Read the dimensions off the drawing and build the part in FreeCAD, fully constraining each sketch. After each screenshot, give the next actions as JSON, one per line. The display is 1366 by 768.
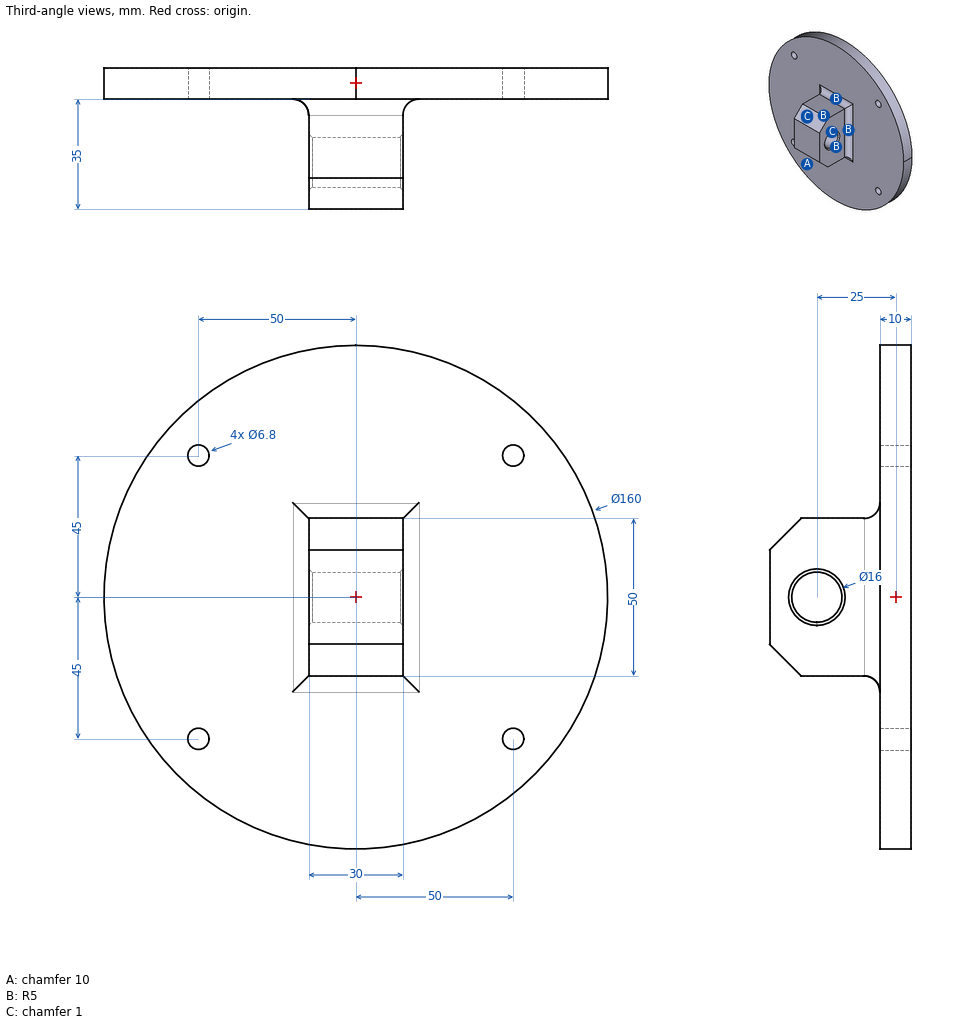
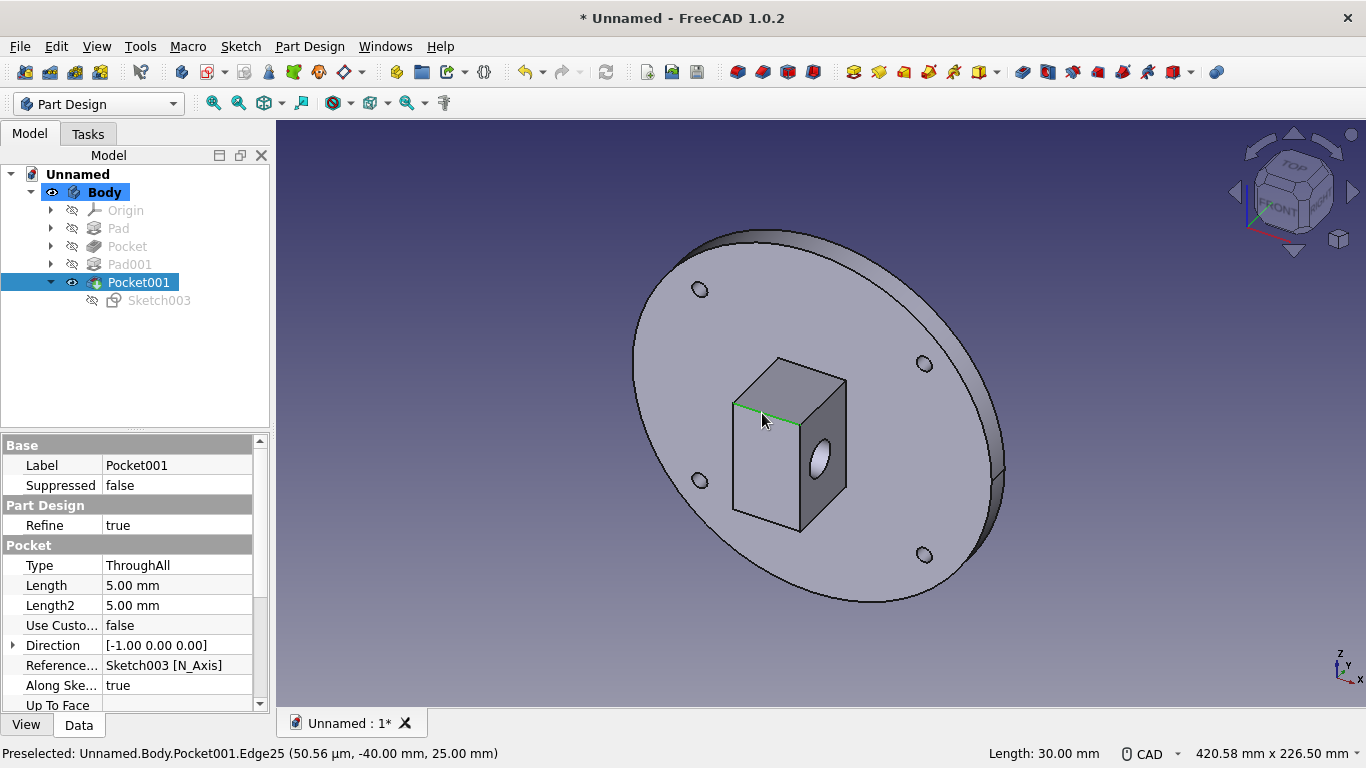
{"action": "key", "text": "0"}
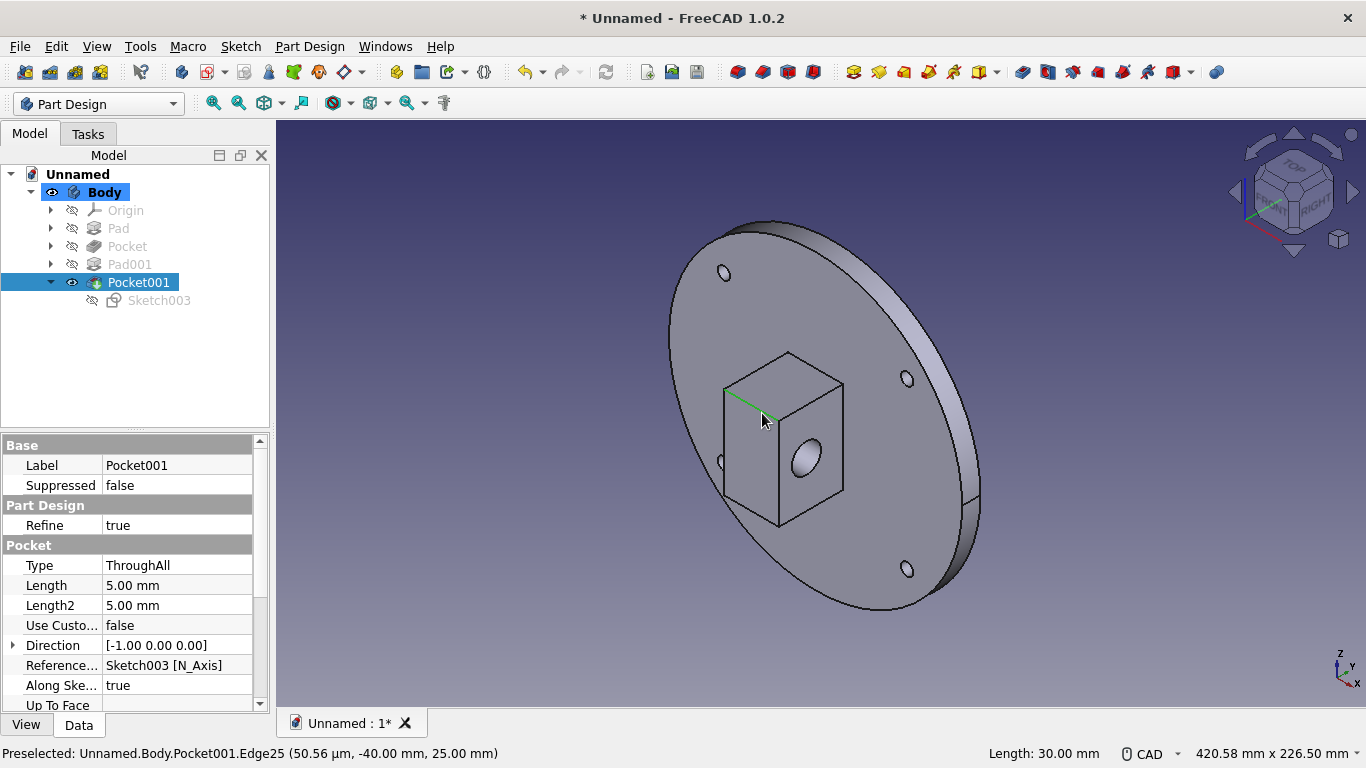
{"action": "key", "text": "v f"}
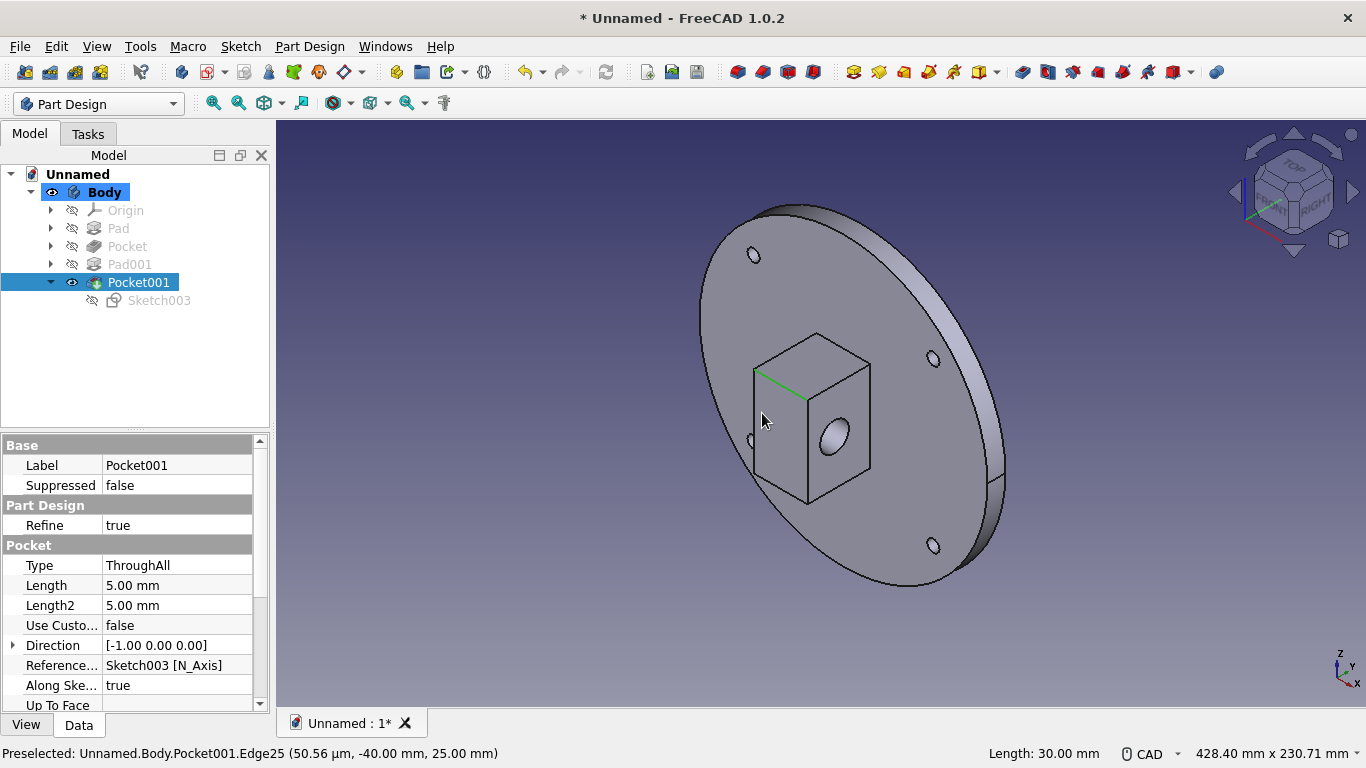
{"action": "key", "text": "2"}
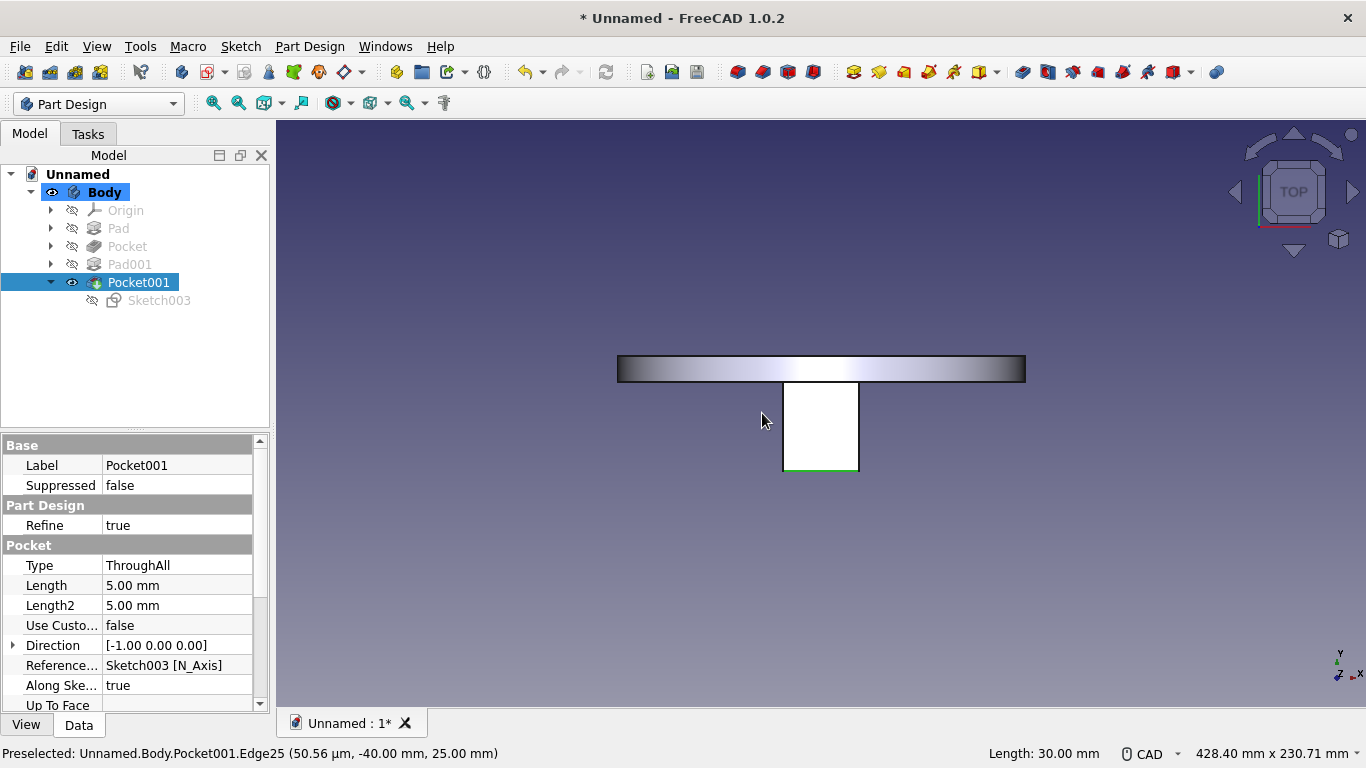
{"action": "key", "text": "v f"}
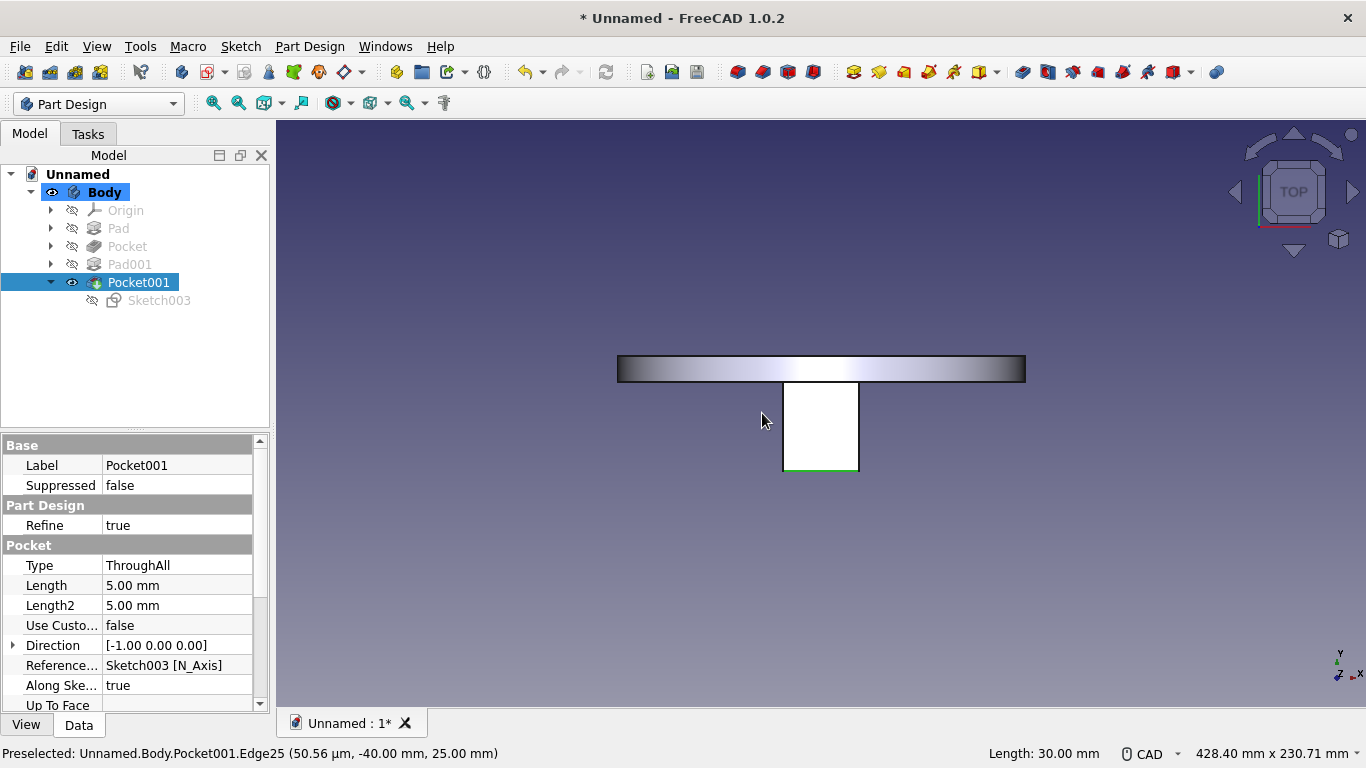
{"action": "key", "text": "1"}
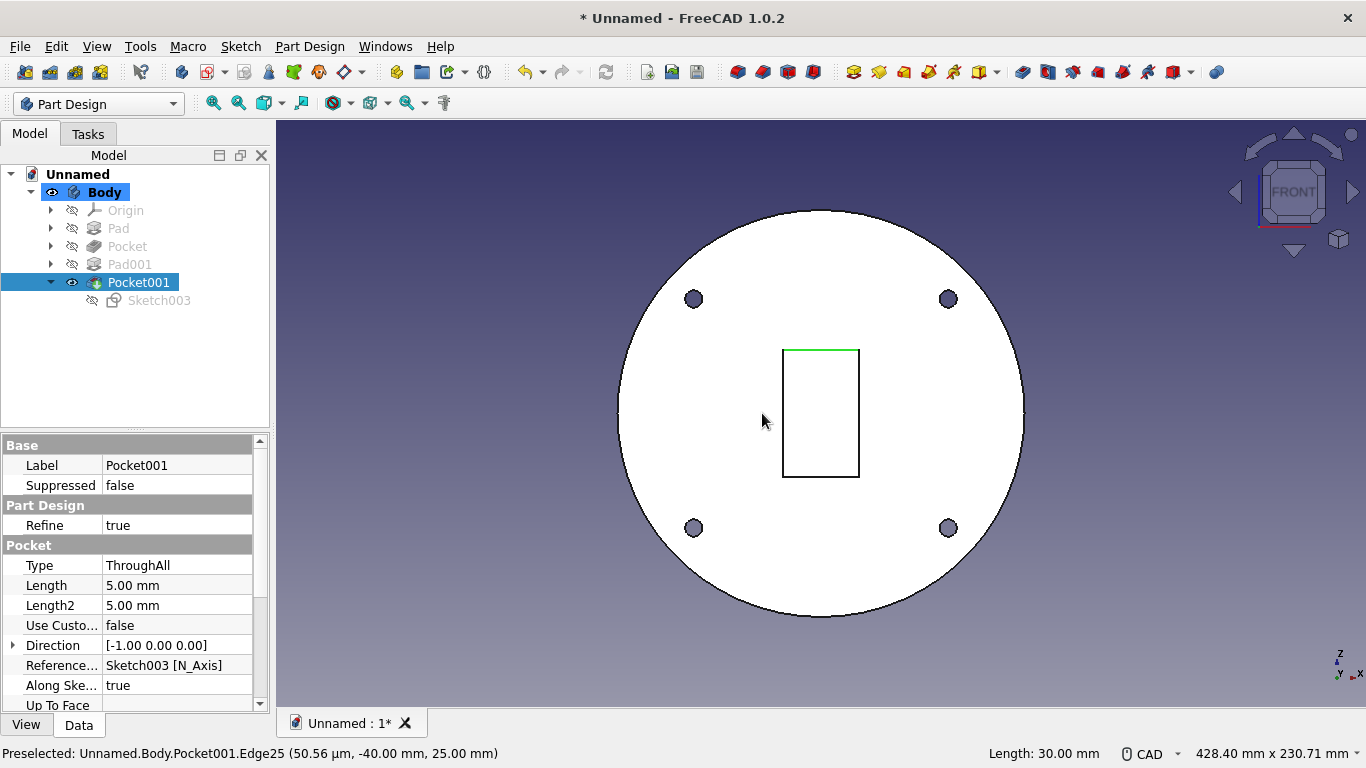
{"action": "key", "text": "3"}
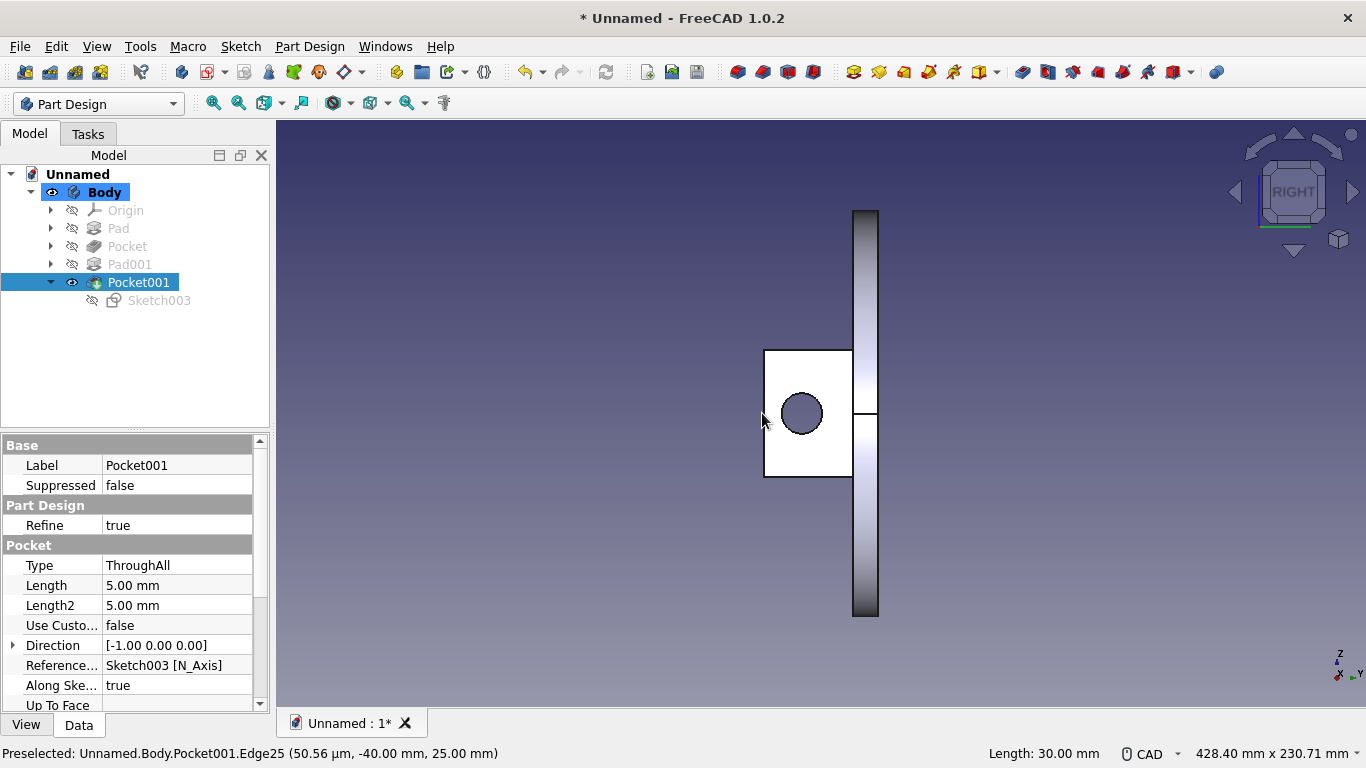
{"action": "key", "text": "5"}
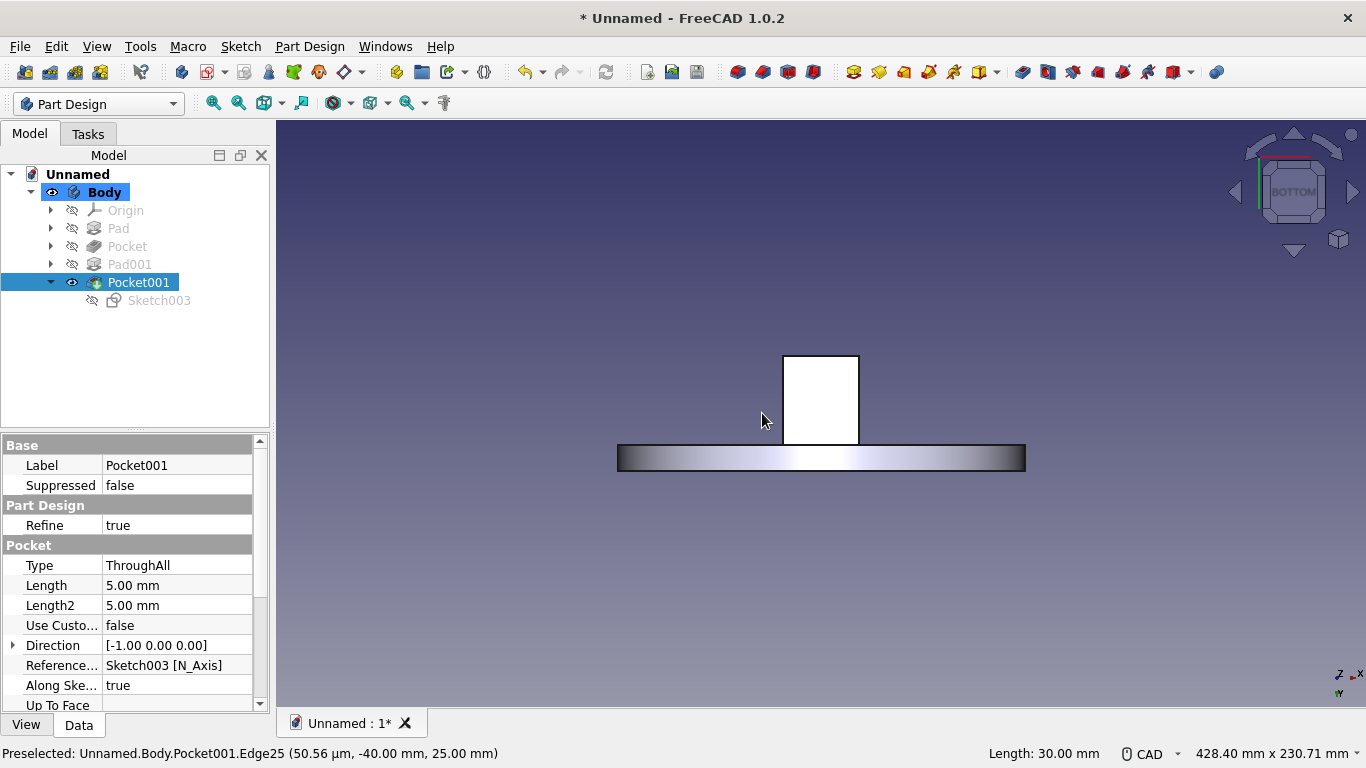
{"action": "key", "text": "v f"}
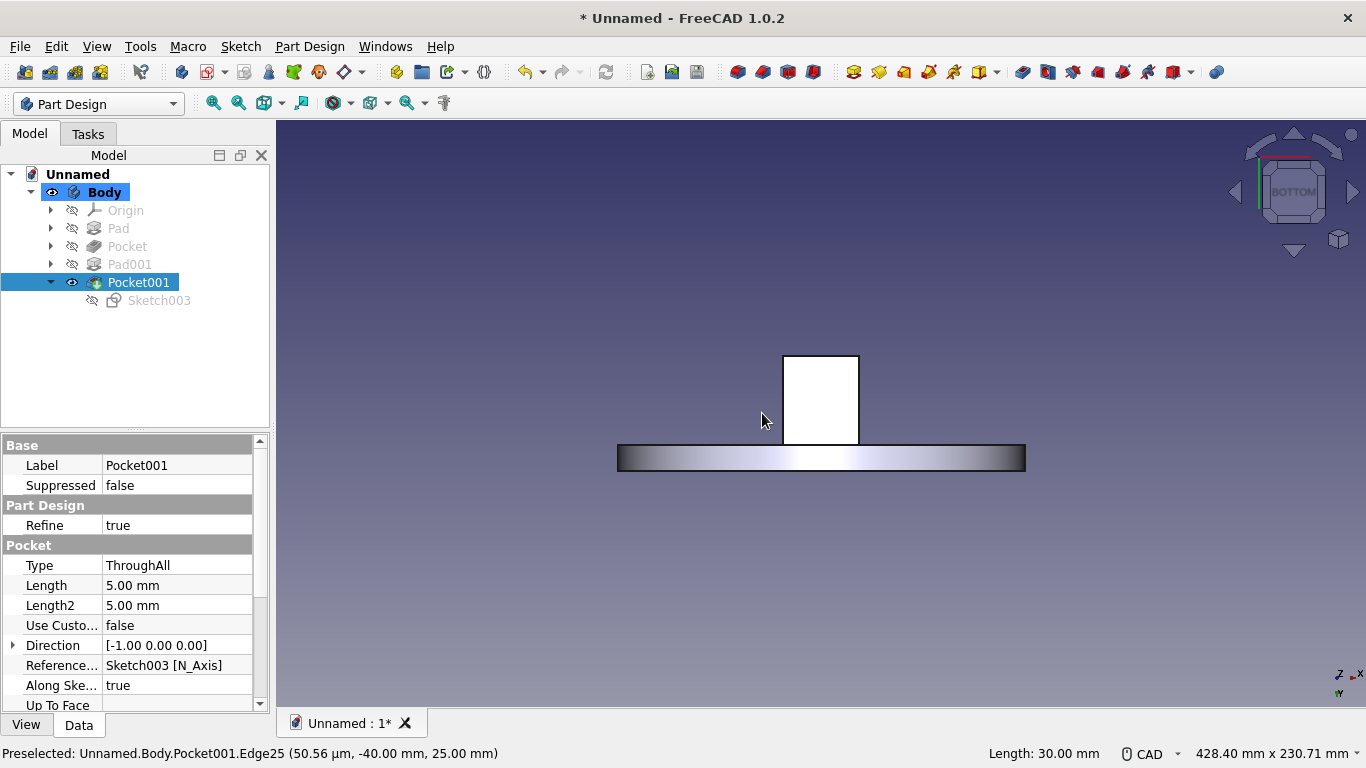
{"action": "left_click", "coordinate": [821, 355], "text": "ctrl"}